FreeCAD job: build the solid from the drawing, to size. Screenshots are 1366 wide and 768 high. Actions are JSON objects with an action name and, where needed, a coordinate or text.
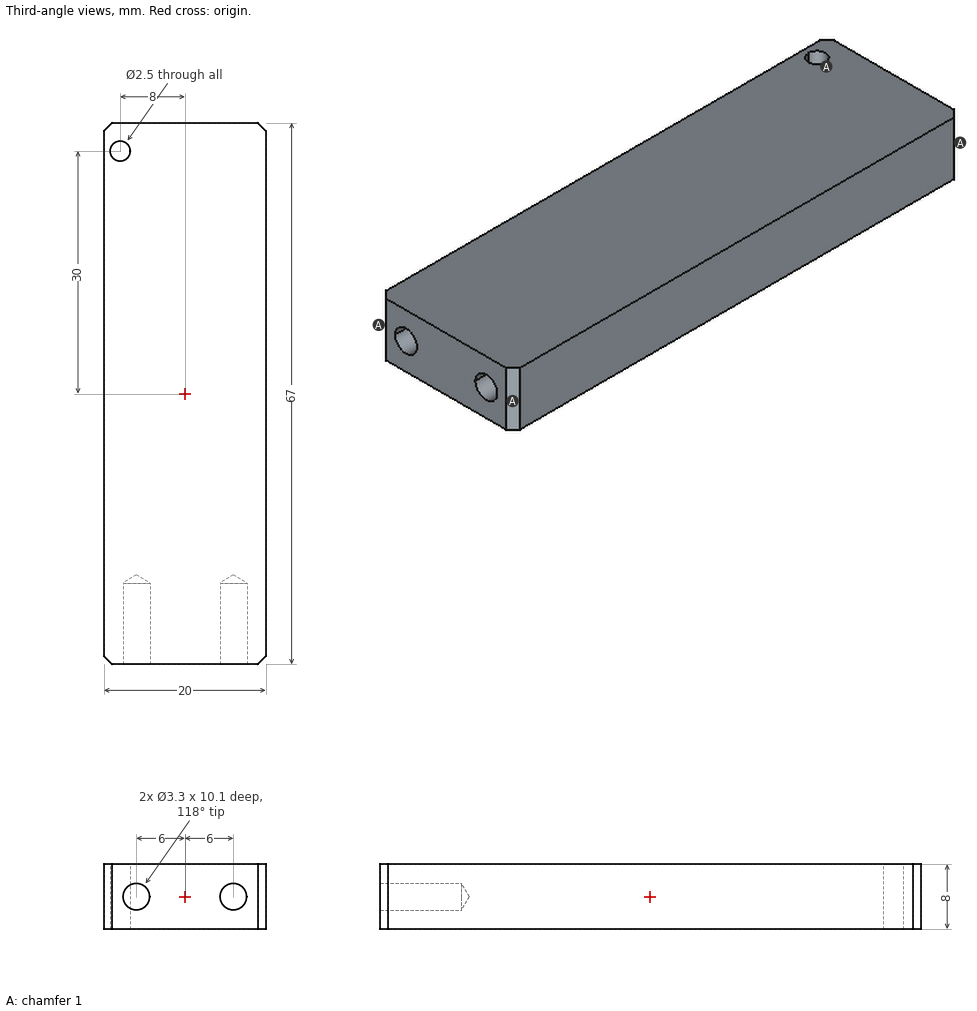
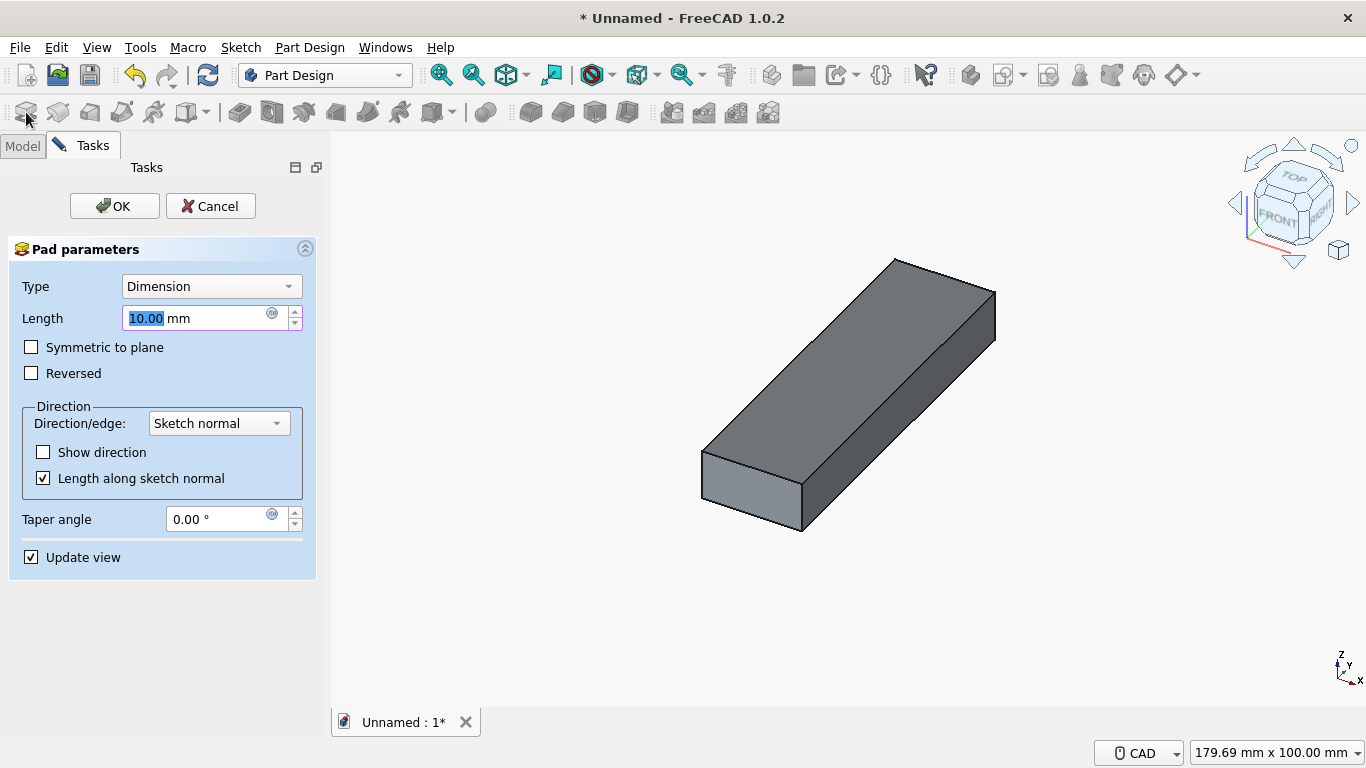
{"action": "type", "text": "8"}
{"action": "key", "text": "Tab"}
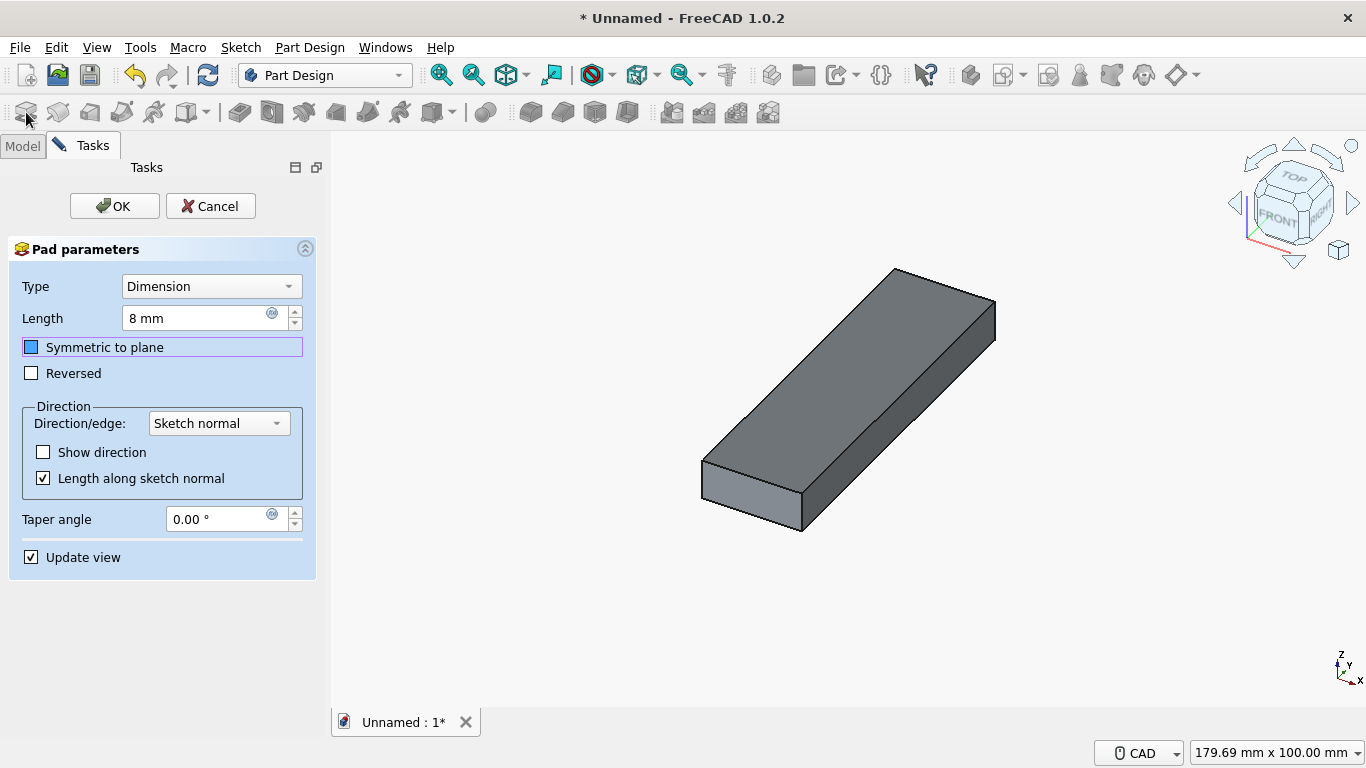
{"action": "left_click", "coordinate": [30, 347]}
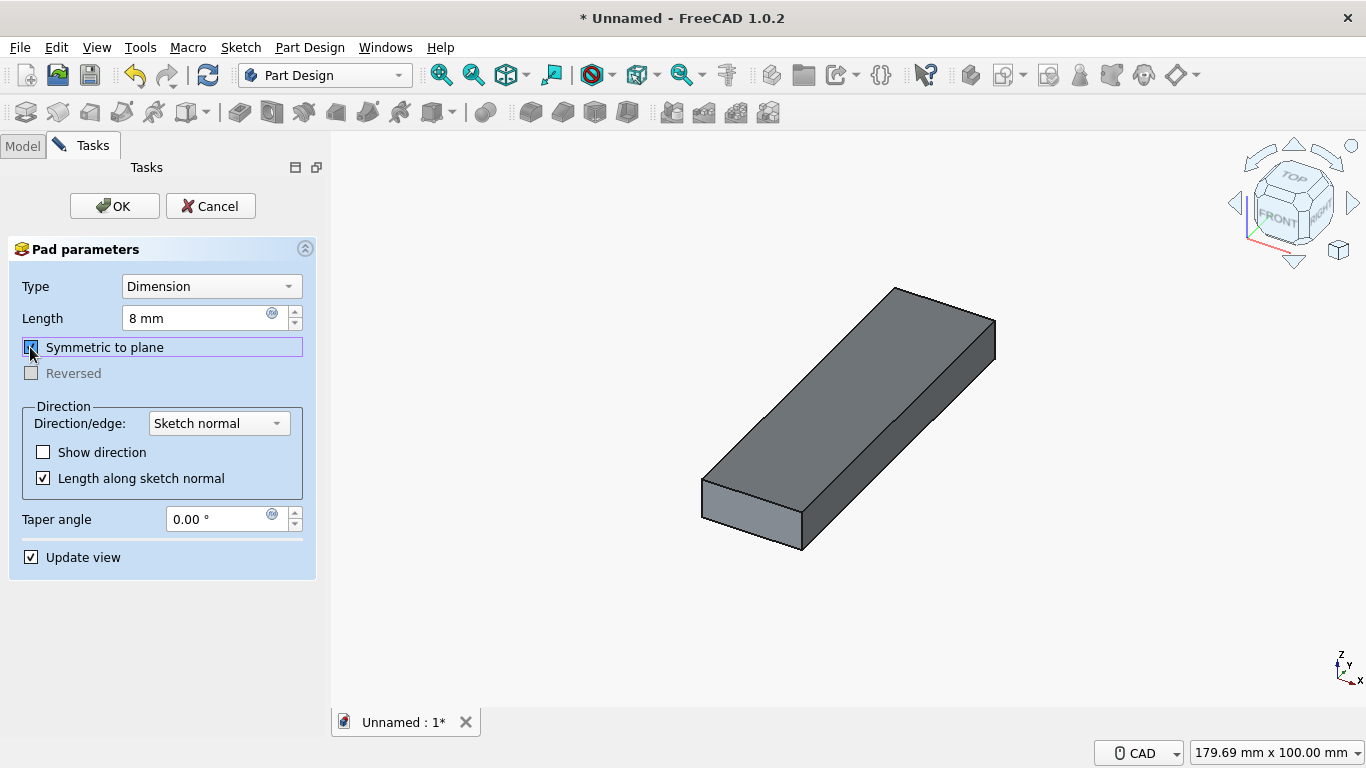
{"action": "left_click", "coordinate": [115, 206]}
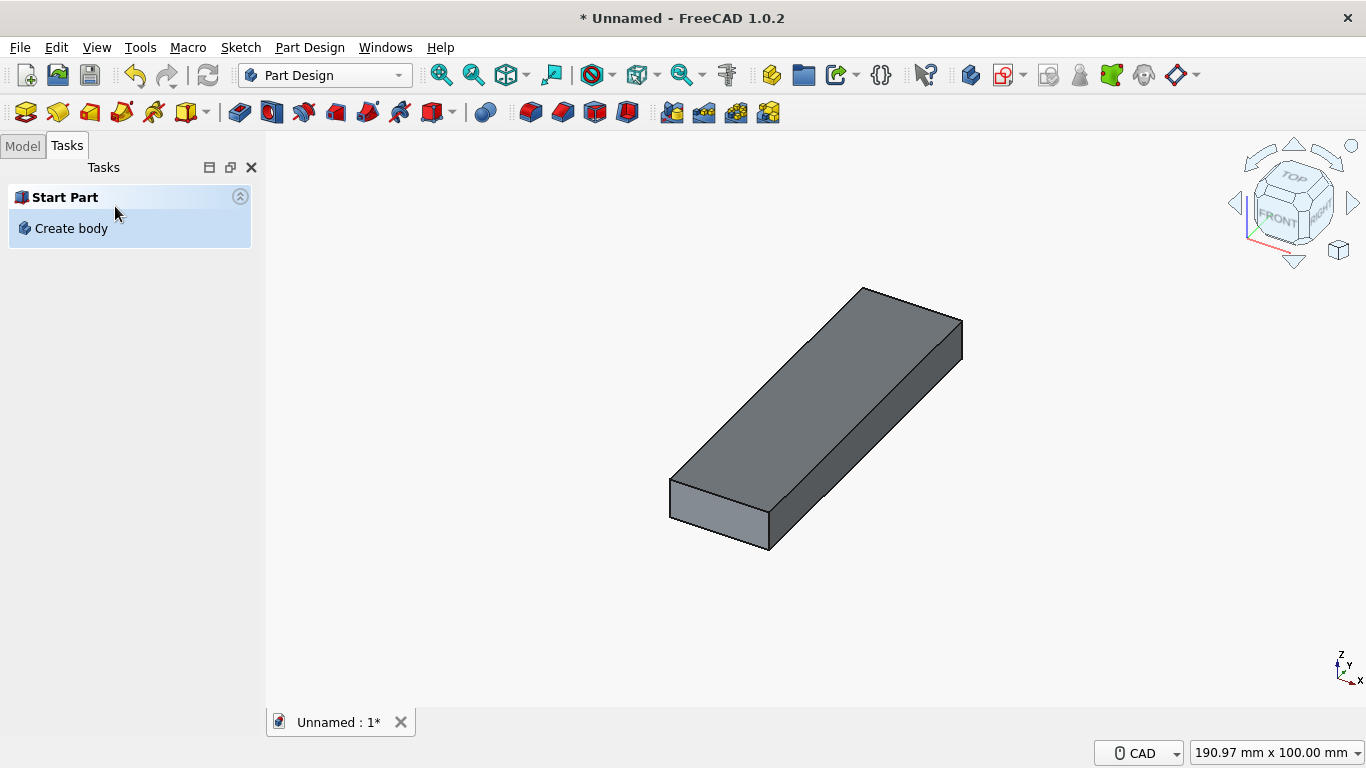
{"action": "key", "text": "5"}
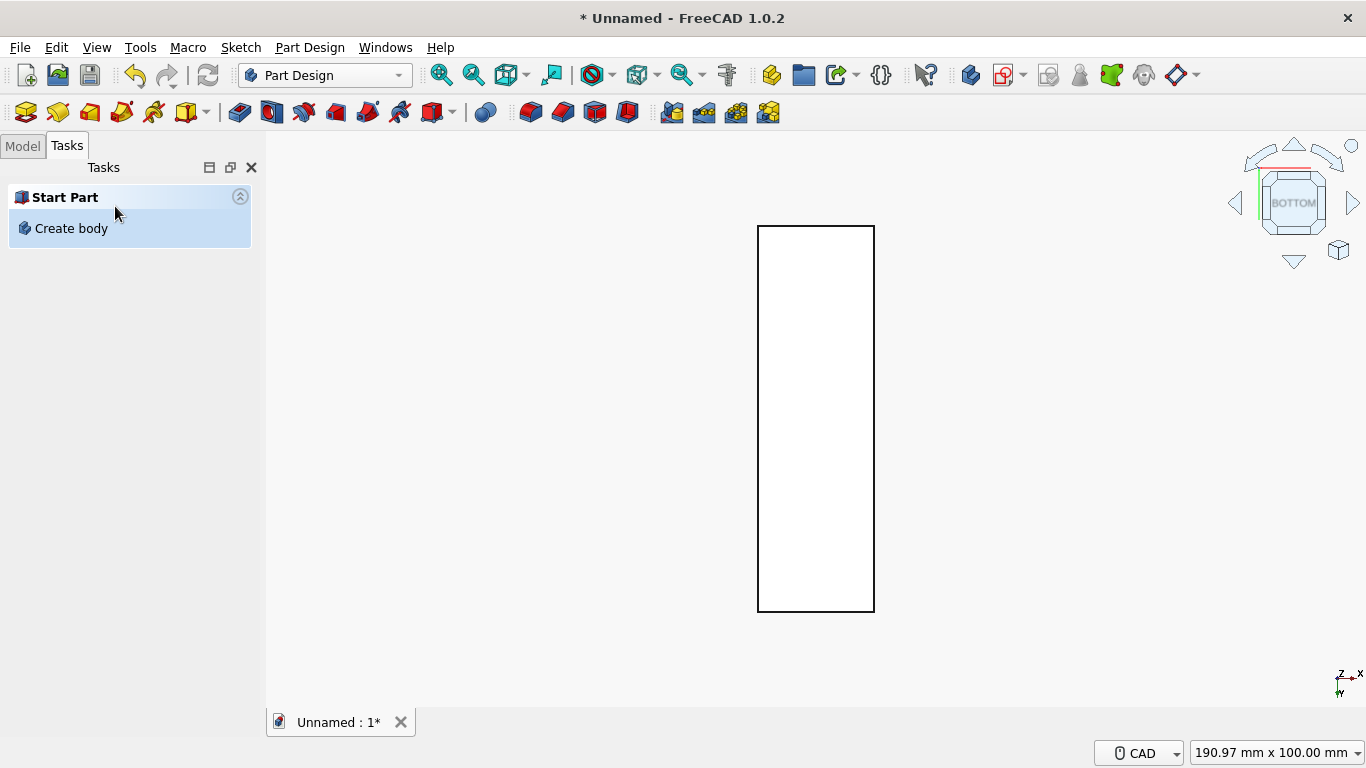
{"action": "left_click", "coordinate": [816, 528]}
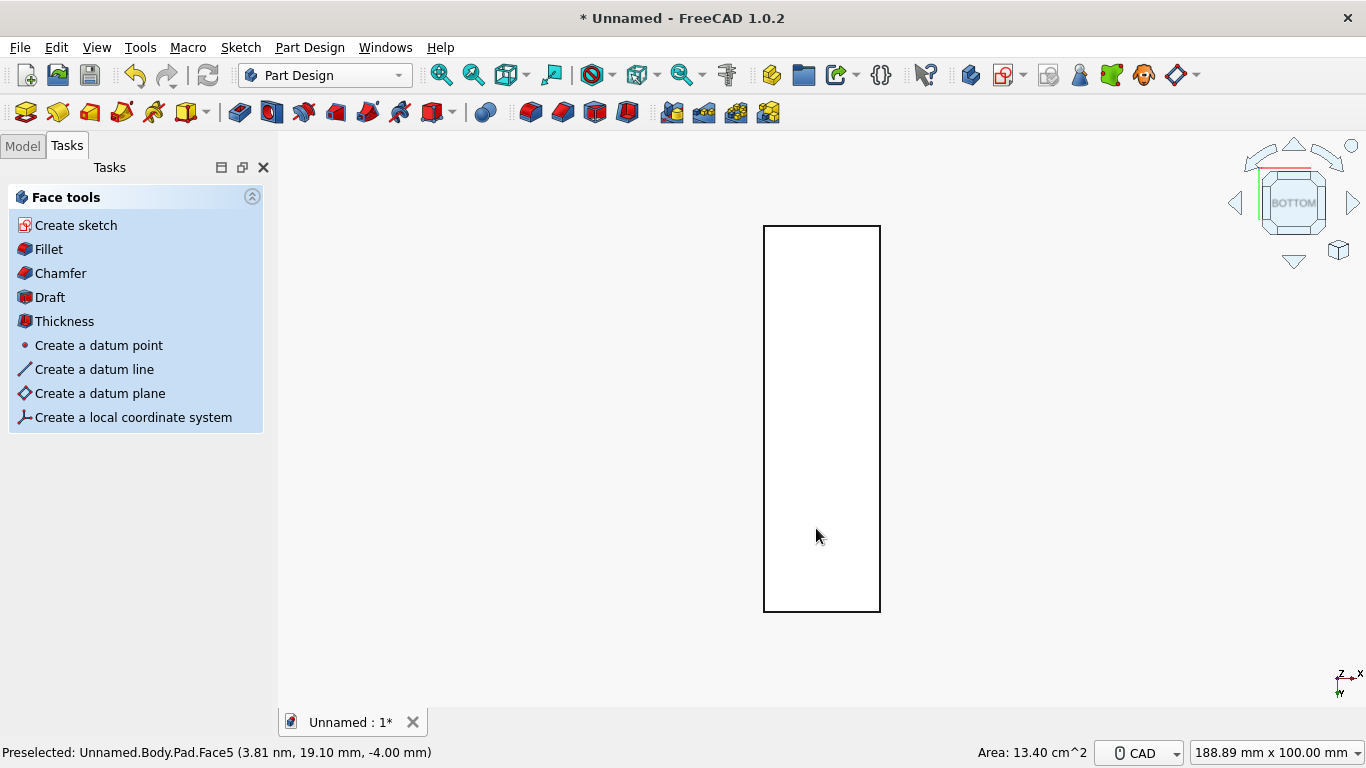
{"action": "left_click", "coordinate": [1004, 76]}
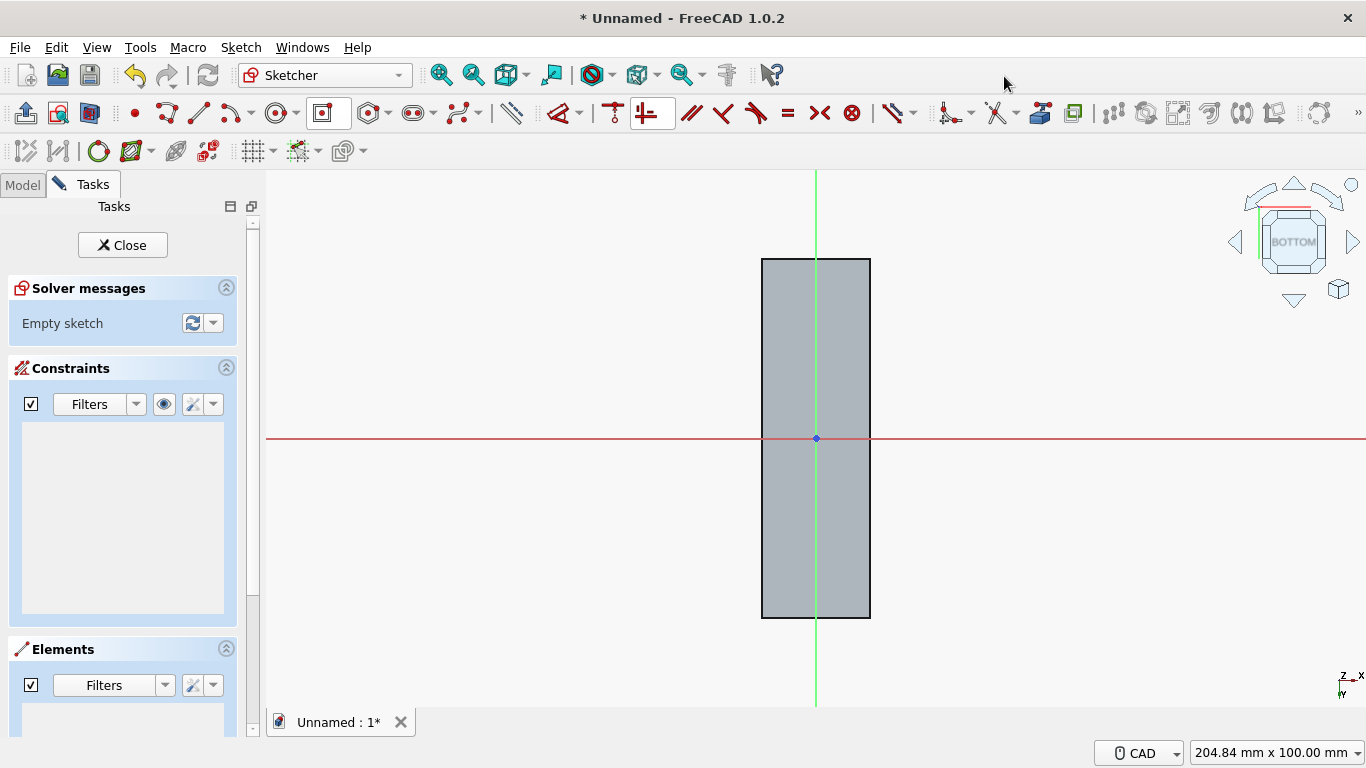
{"action": "scroll", "coordinate": [774, 608], "scroll_direction": "up", "scroll_amount": 15}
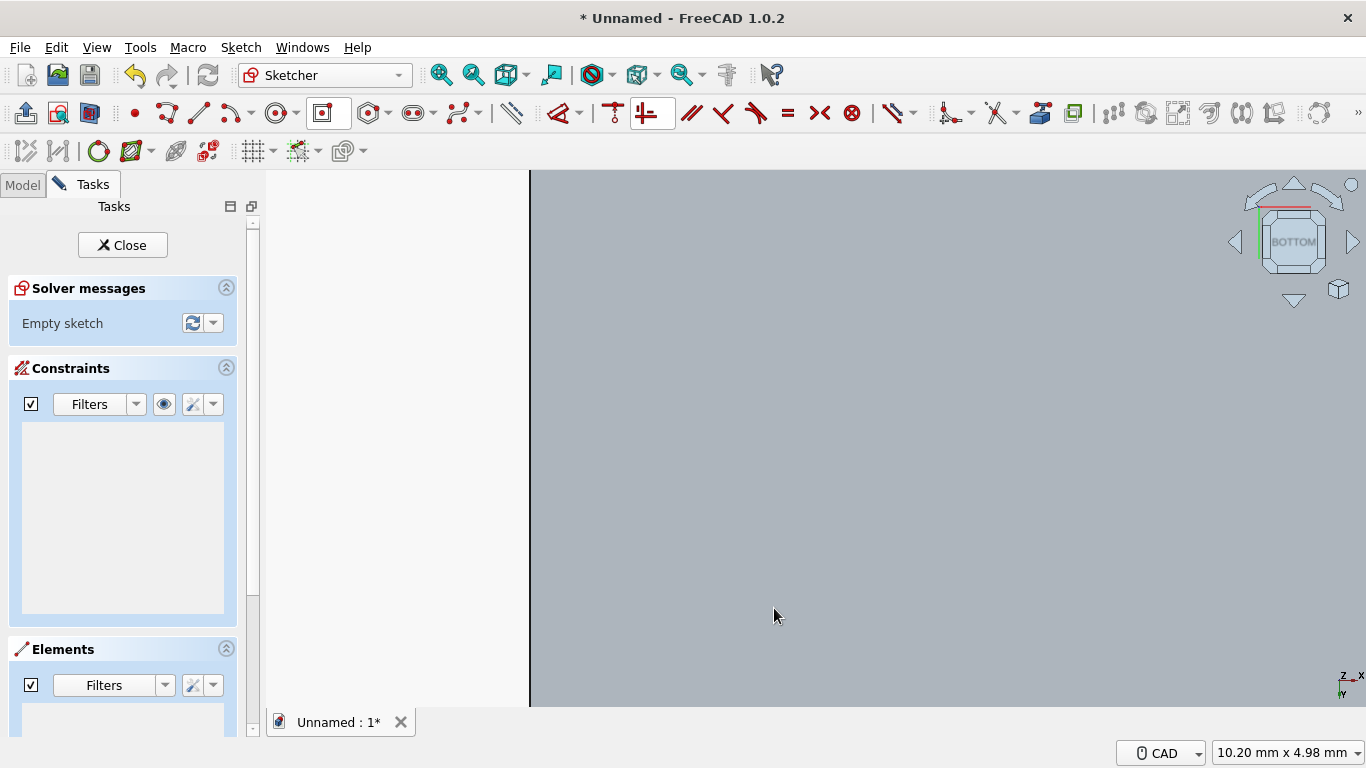
{"action": "key", "text": "g c"}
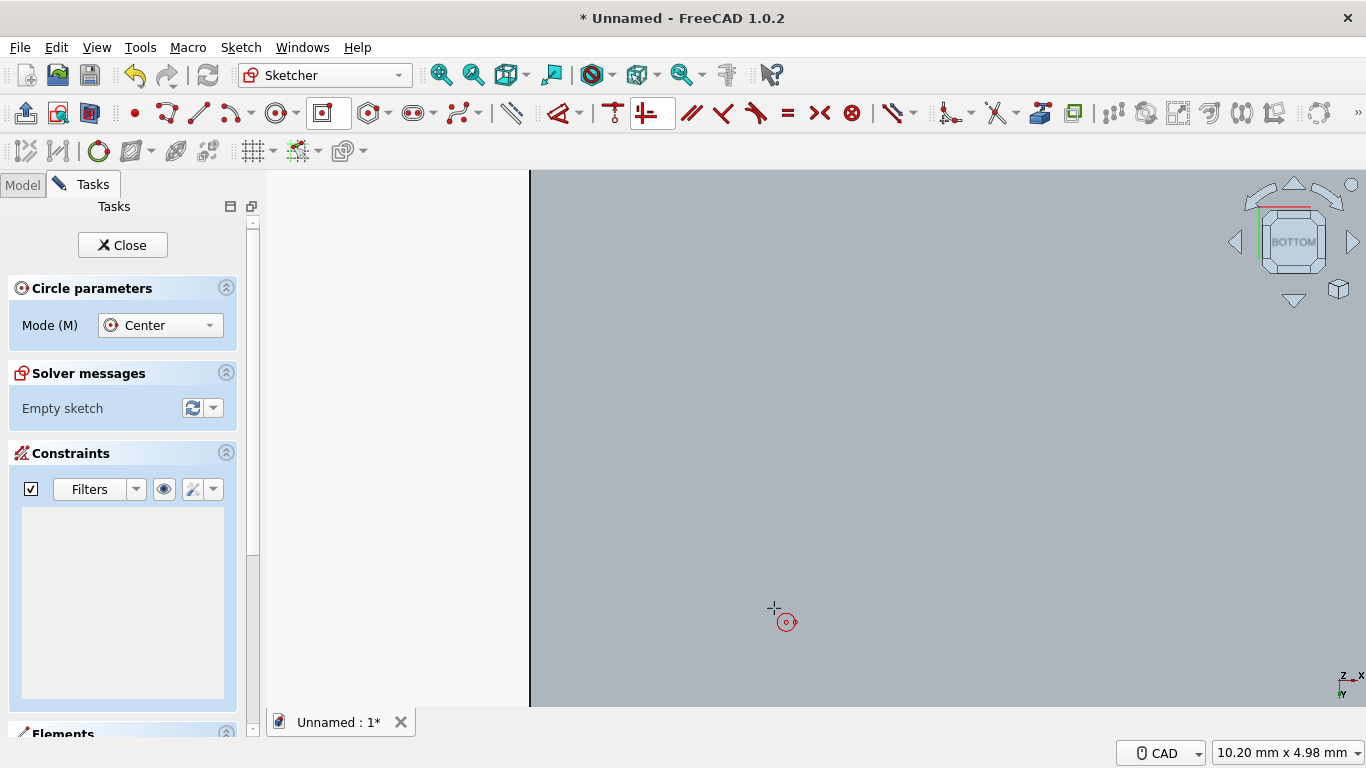
{"action": "left_click", "coordinate": [746, 424]}
{"action": "mouse_move", "coordinate": [841, 328]}